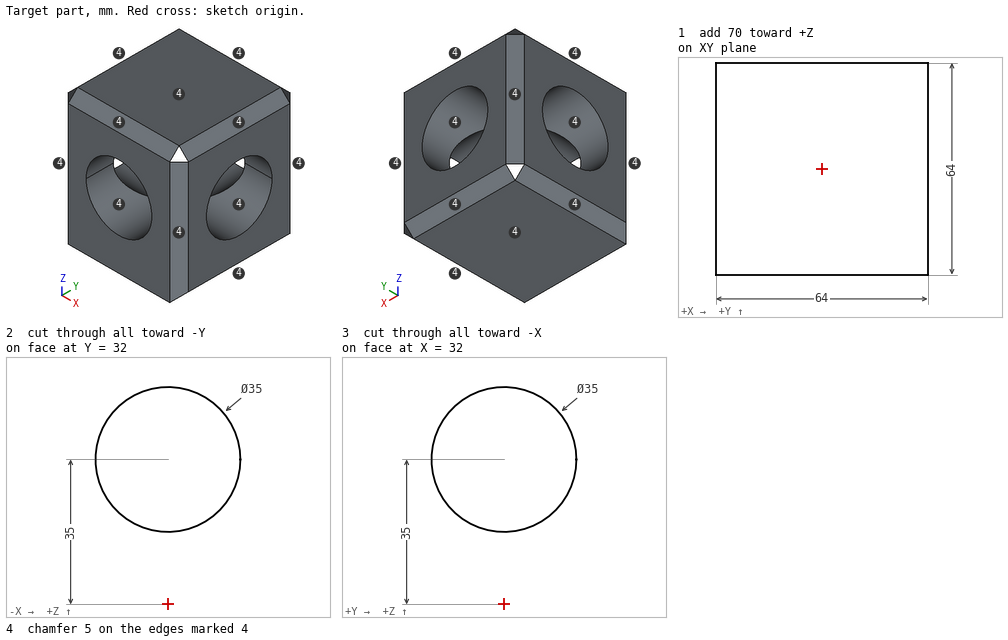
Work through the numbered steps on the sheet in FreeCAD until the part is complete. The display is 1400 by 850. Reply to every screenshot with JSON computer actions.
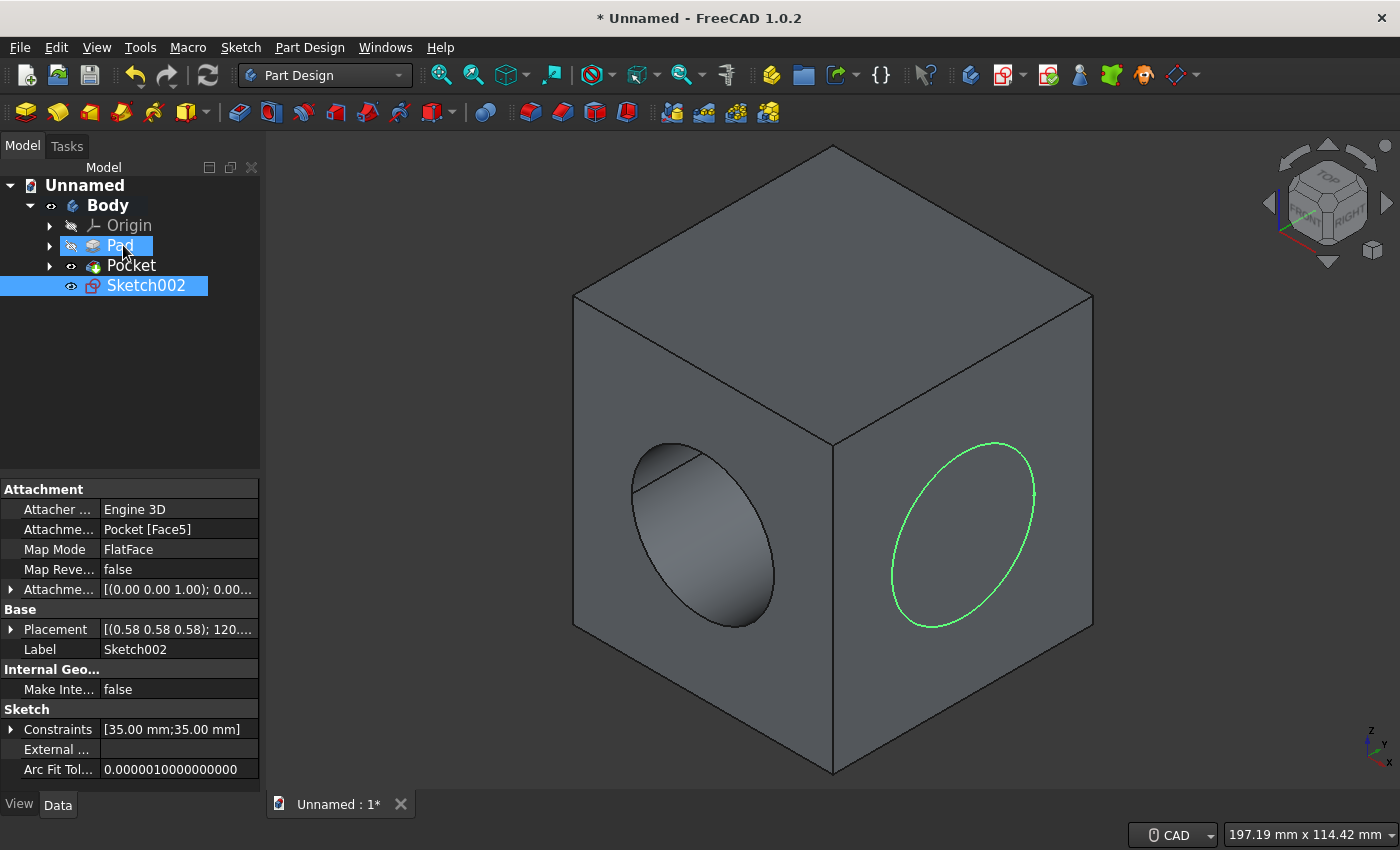
{"action": "left_click", "coordinate": [240, 112]}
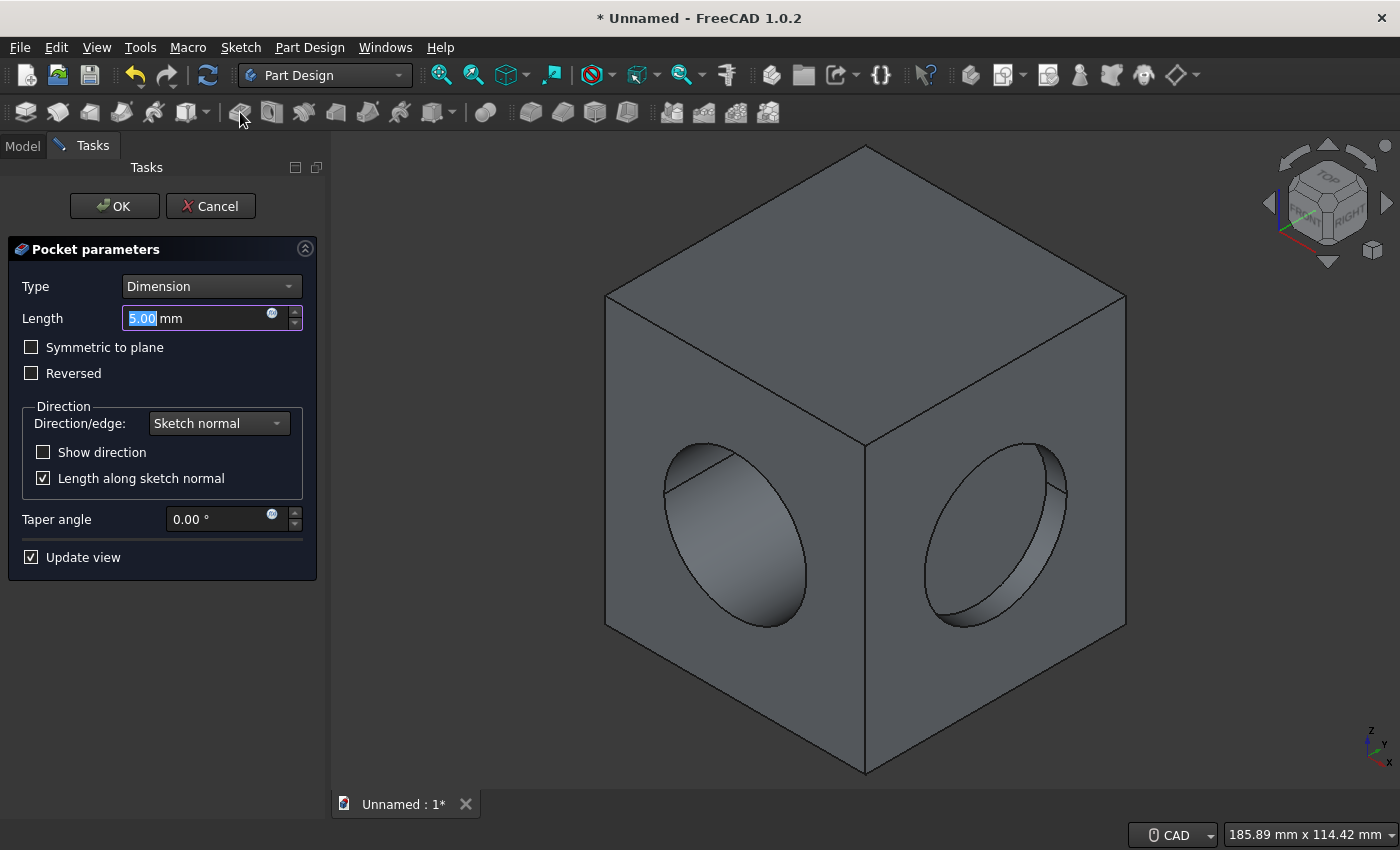
{"action": "left_click", "coordinate": [212, 286]}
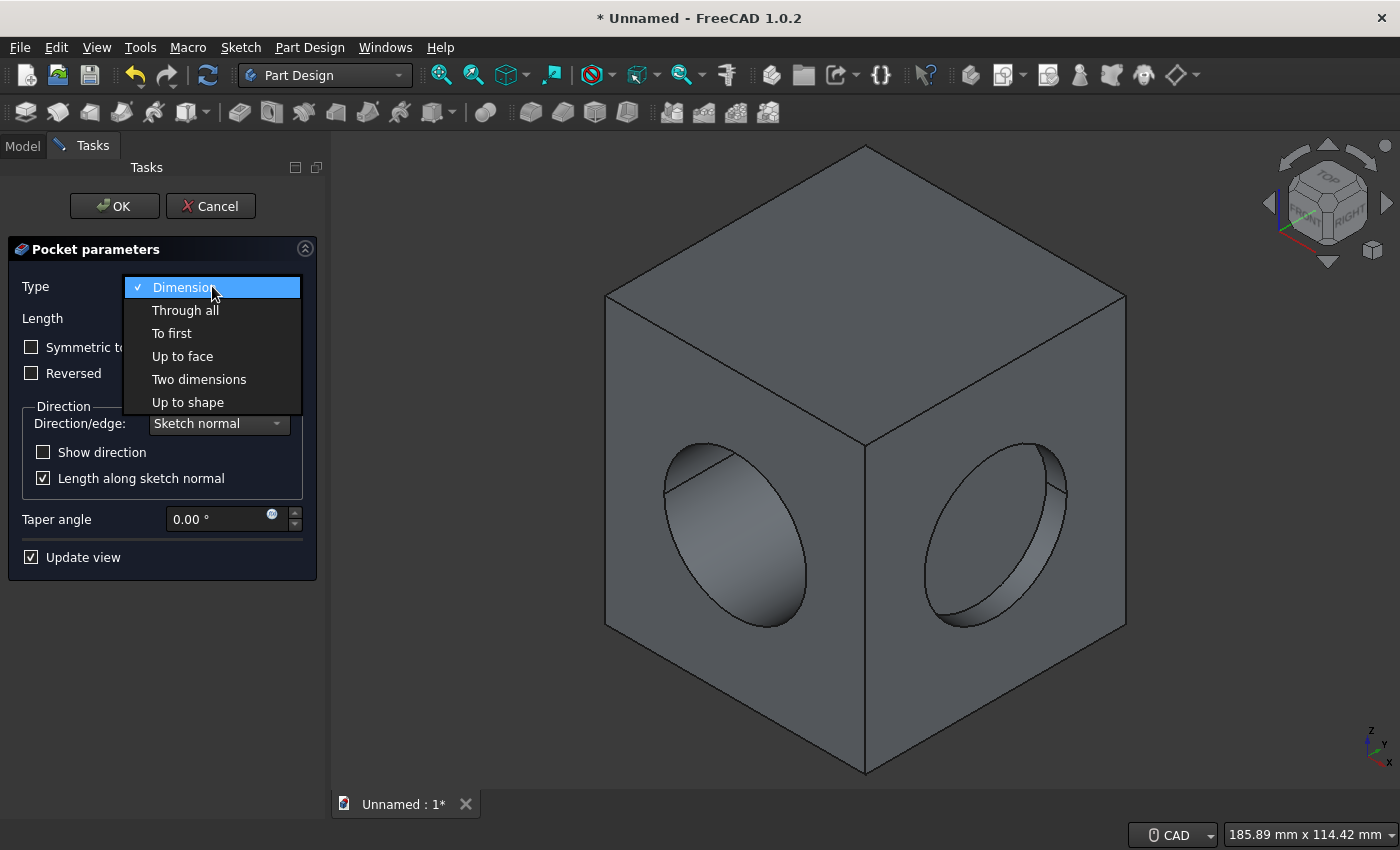
{"action": "left_click", "coordinate": [212, 310]}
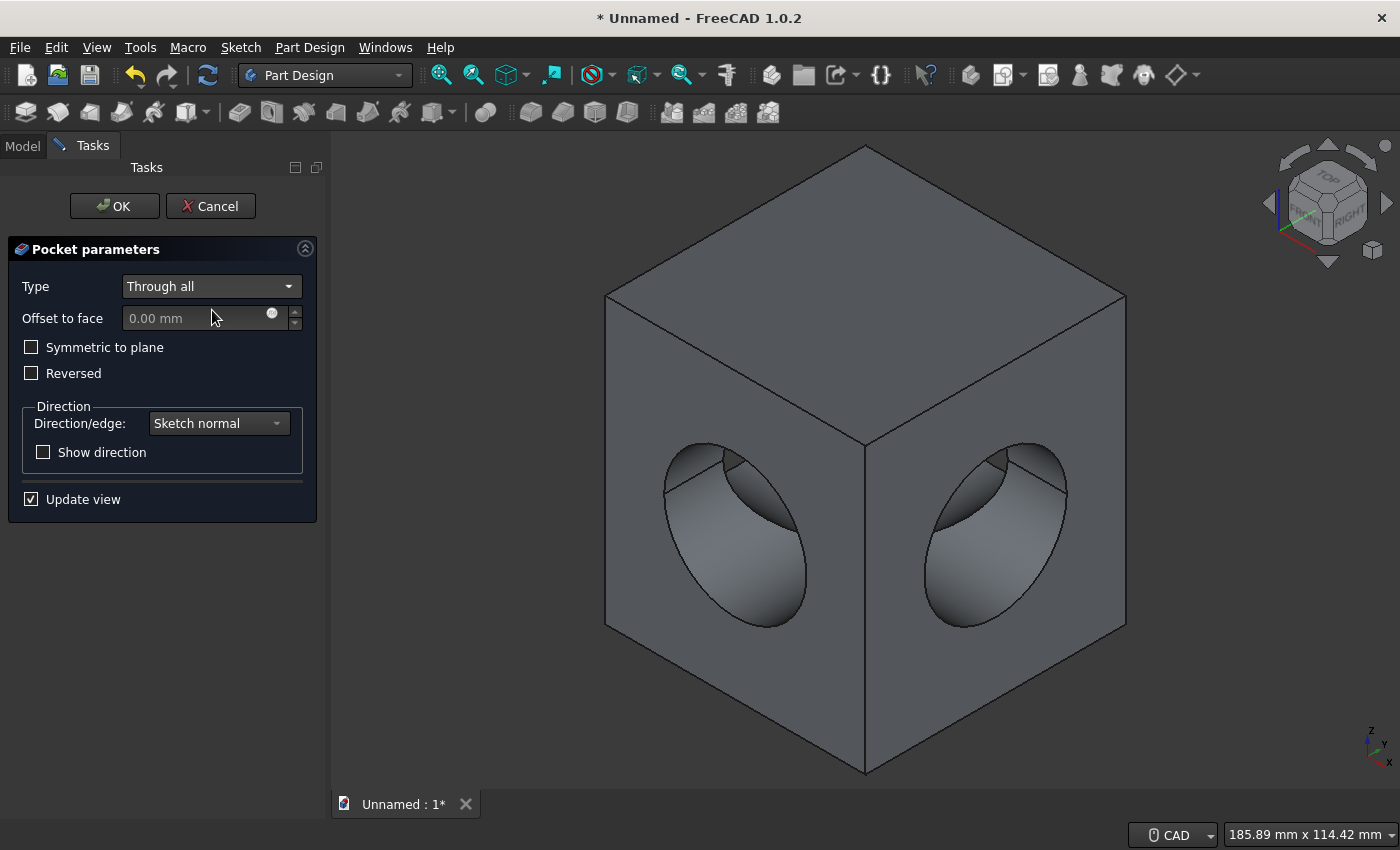
{"action": "left_click", "coordinate": [115, 206]}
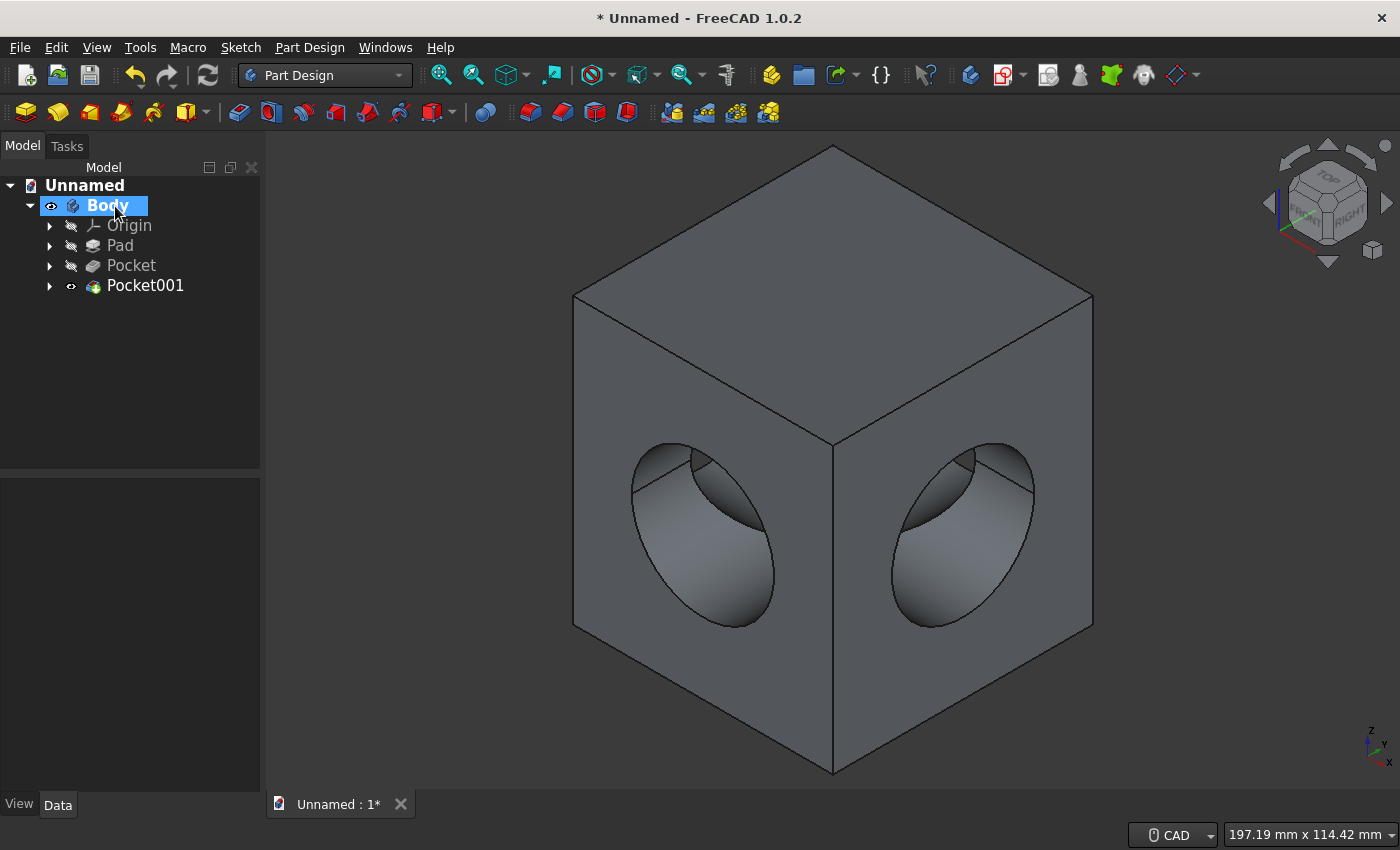
{"action": "left_click", "coordinate": [833, 295]}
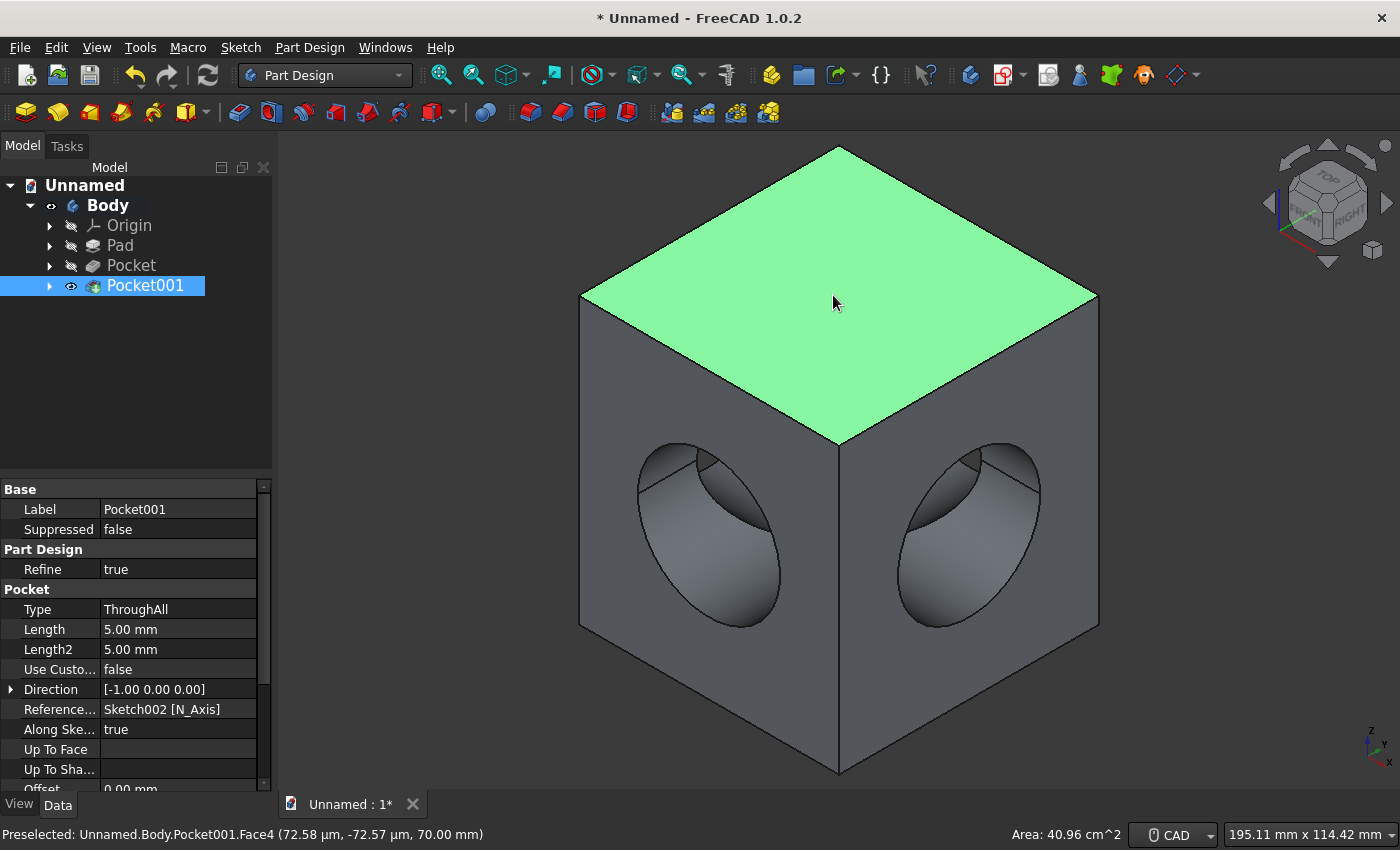
{"action": "left_click", "coordinate": [839, 609], "text": "ctrl"}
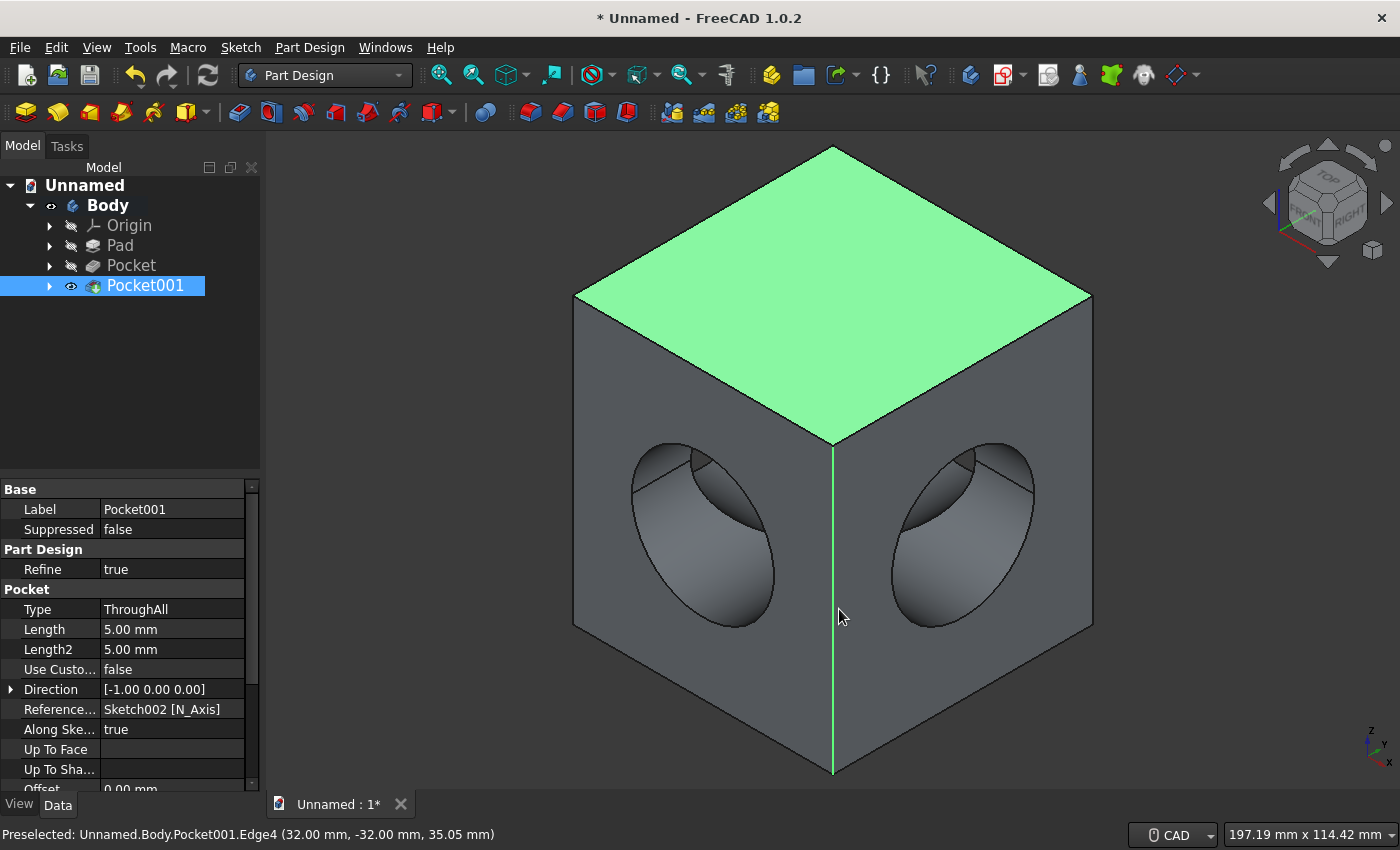
{"action": "key", "text": "2"}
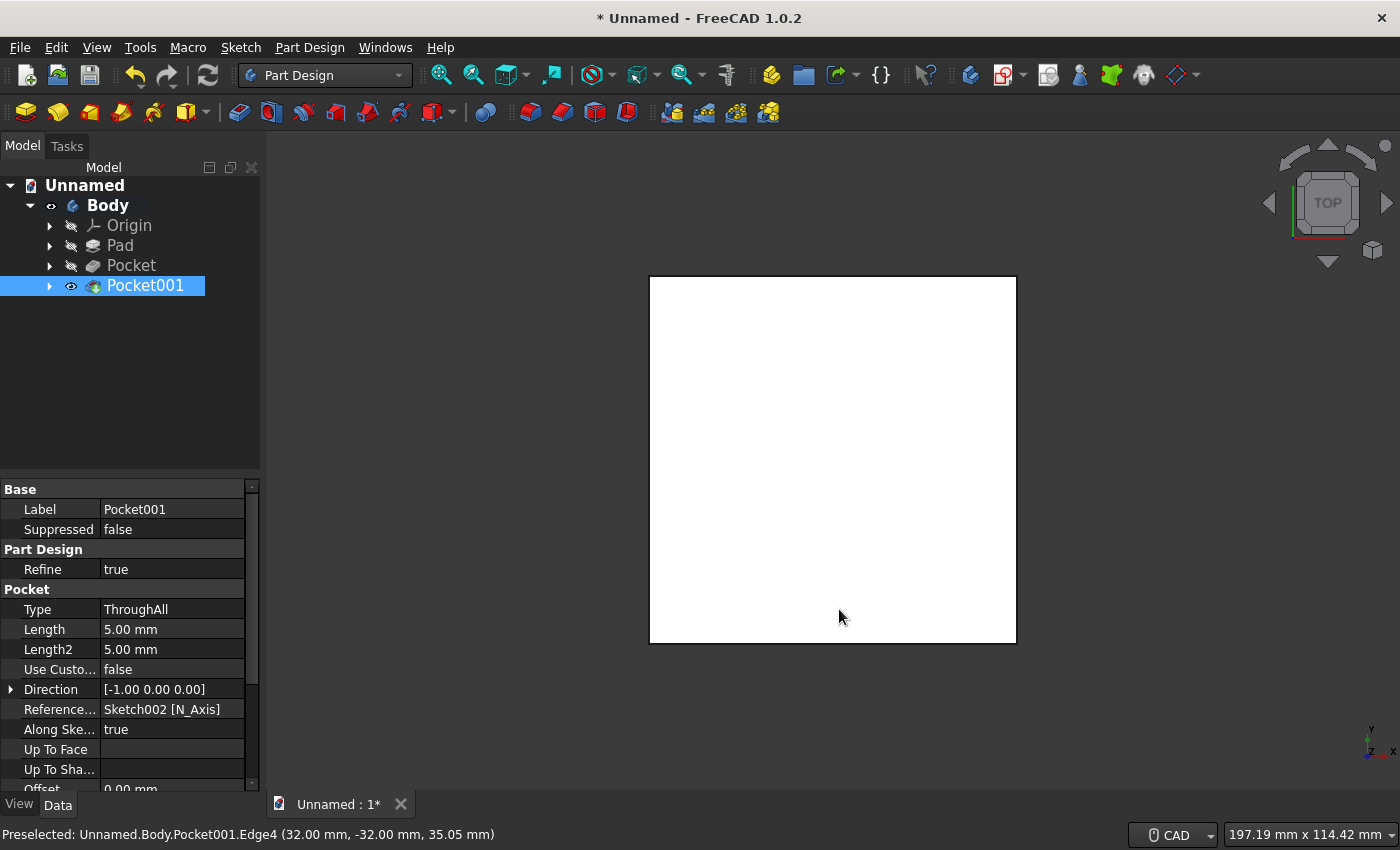
{"action": "key", "text": "0"}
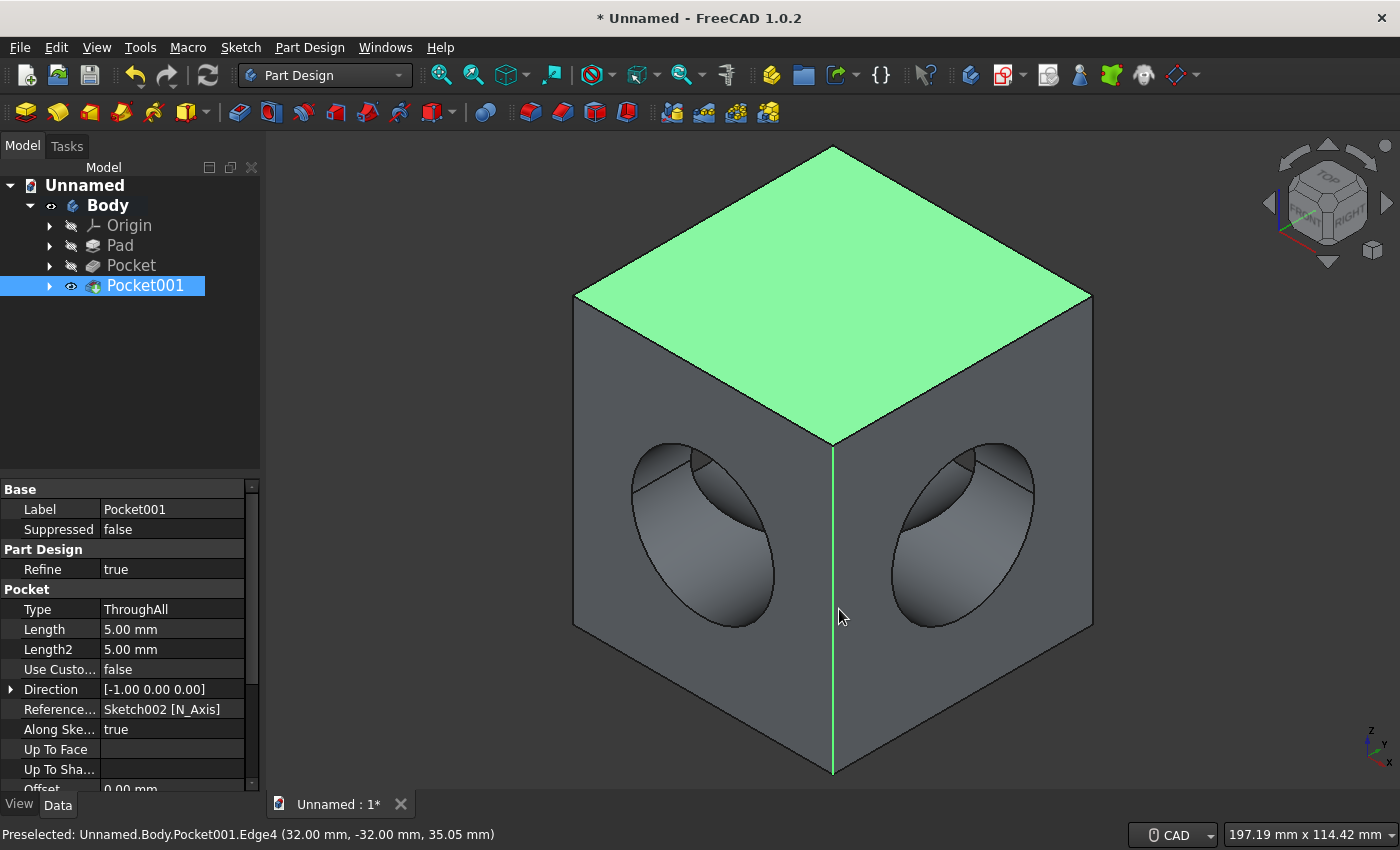
{"action": "key", "text": "1"}